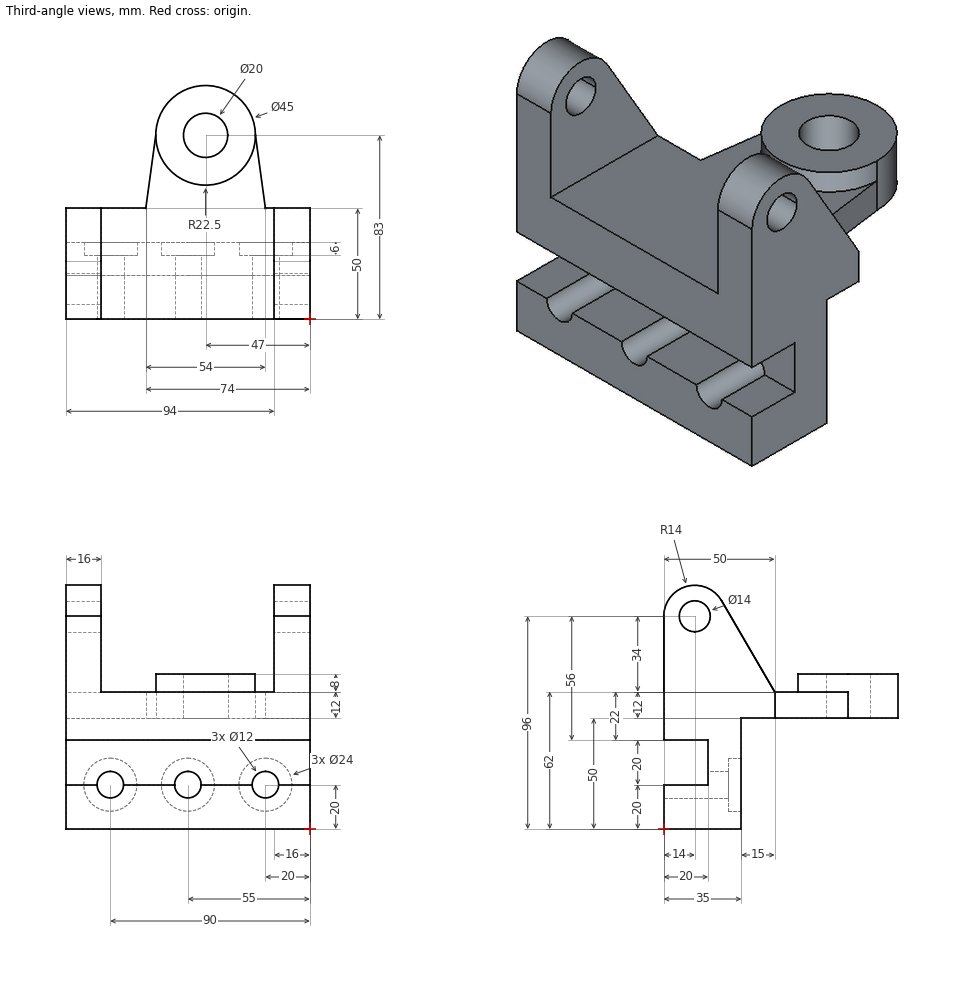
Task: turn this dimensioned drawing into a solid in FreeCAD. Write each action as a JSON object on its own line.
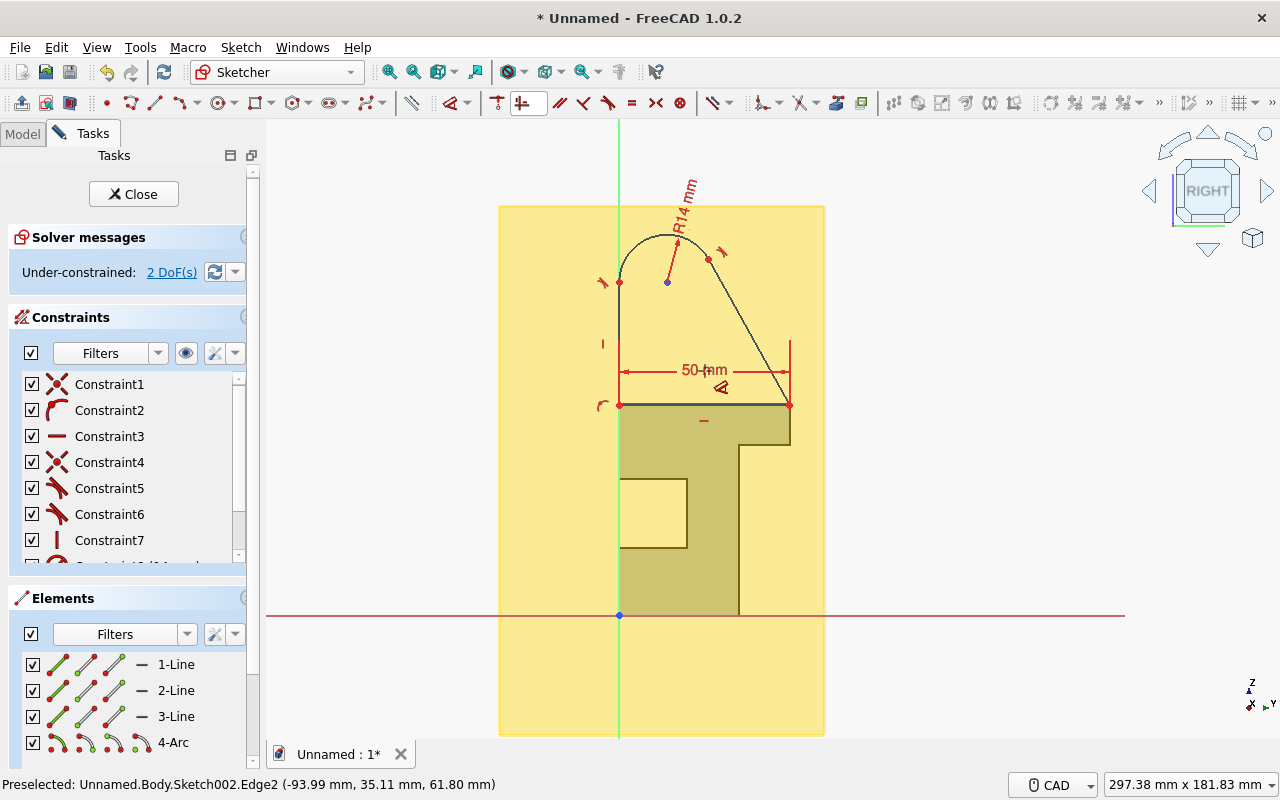
{"action": "left_click", "coordinate": [619, 368]}
{"action": "left_click", "coordinate": [585, 344]}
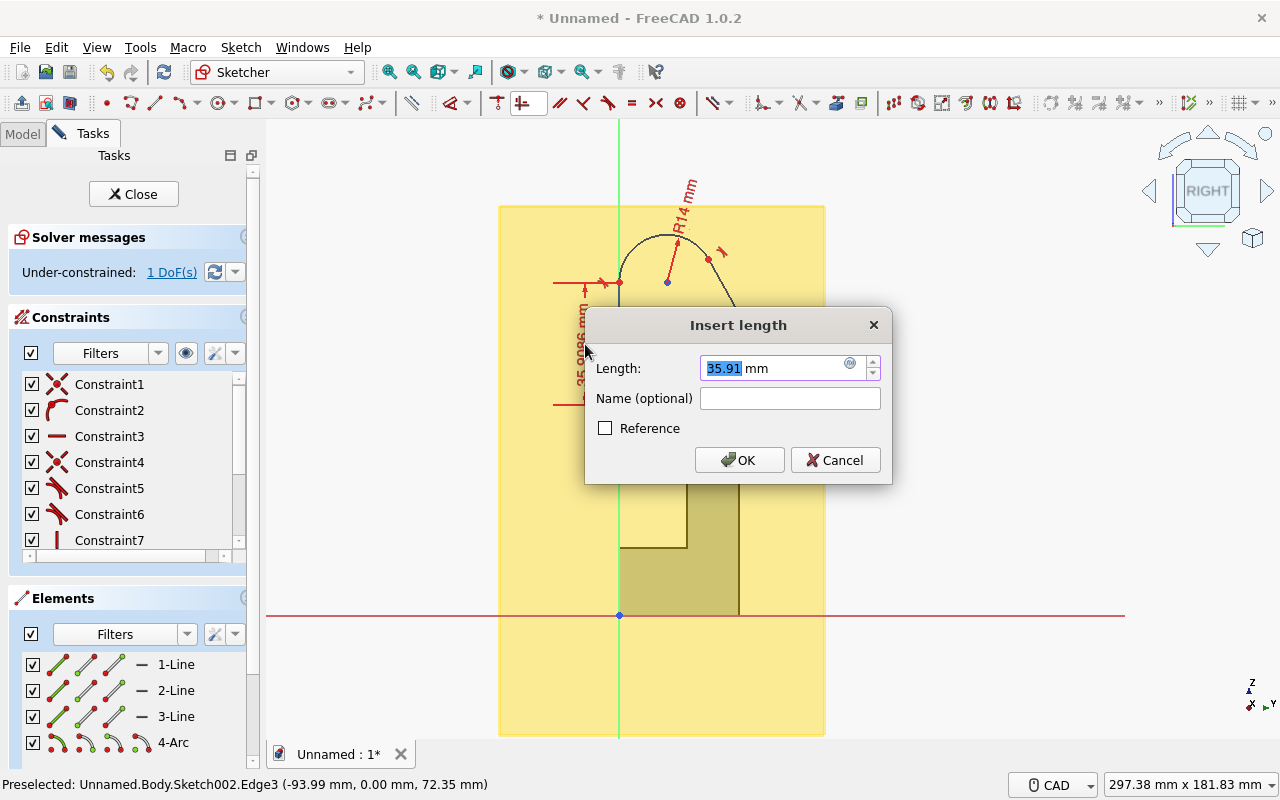
{"action": "type", "text": "34"}
{"action": "key", "text": "Return"}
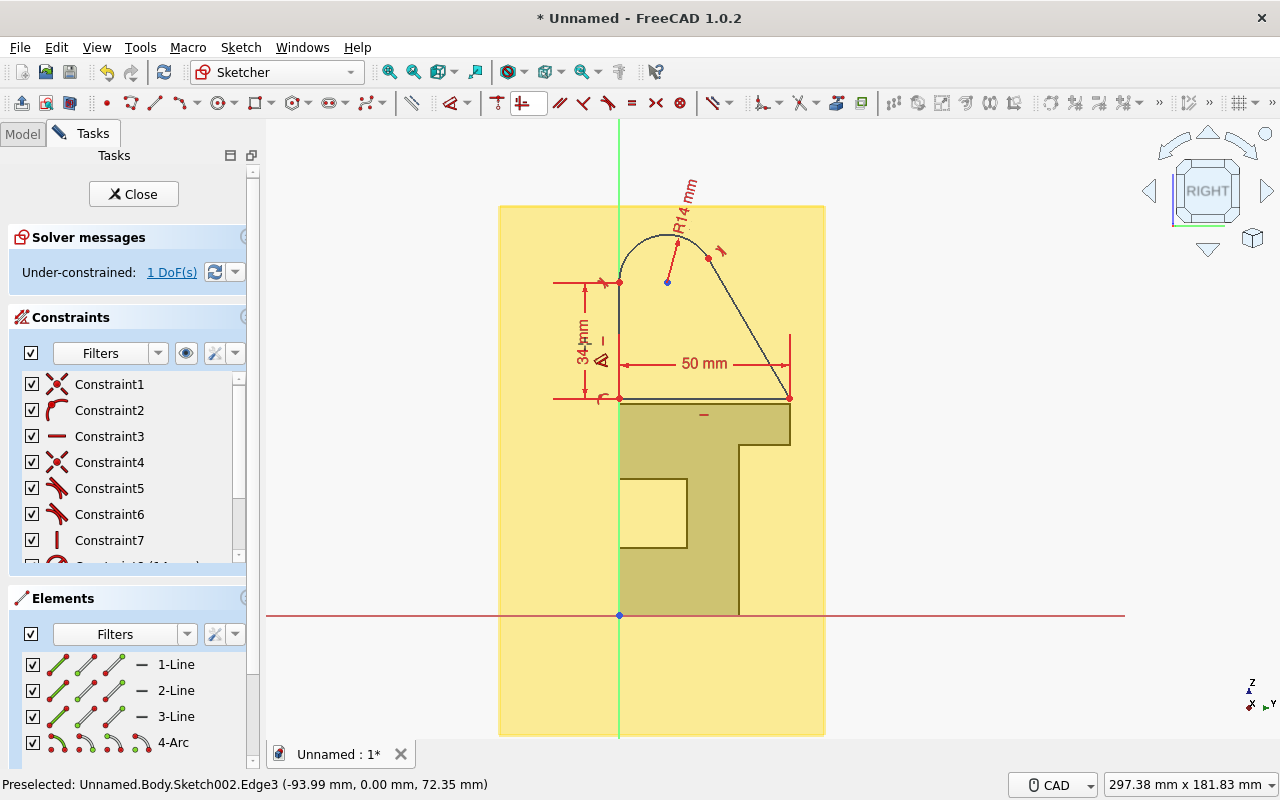
{"action": "left_click", "coordinate": [790, 399]}
{"action": "left_click", "coordinate": [824, 507]}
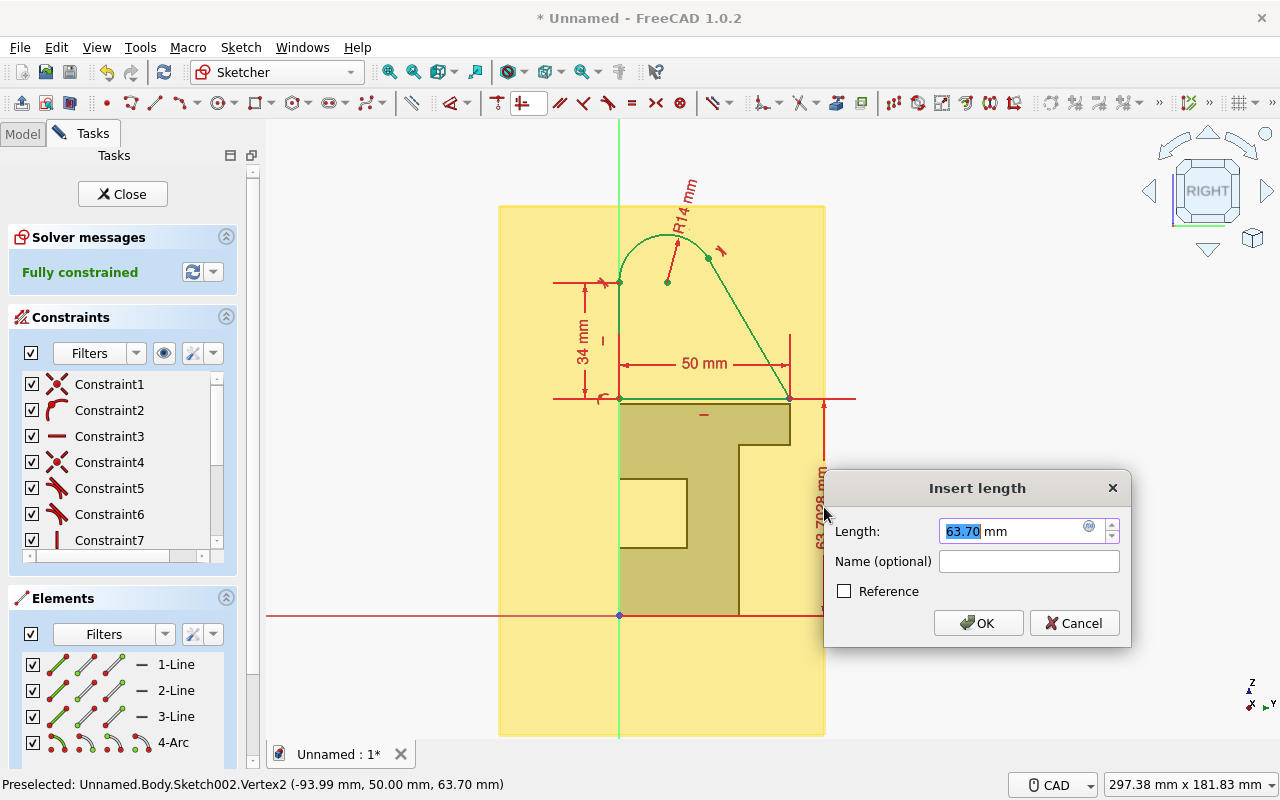
{"action": "type", "text": "62"}
{"action": "key", "text": "Return"}
{"action": "key", "text": "Escape"}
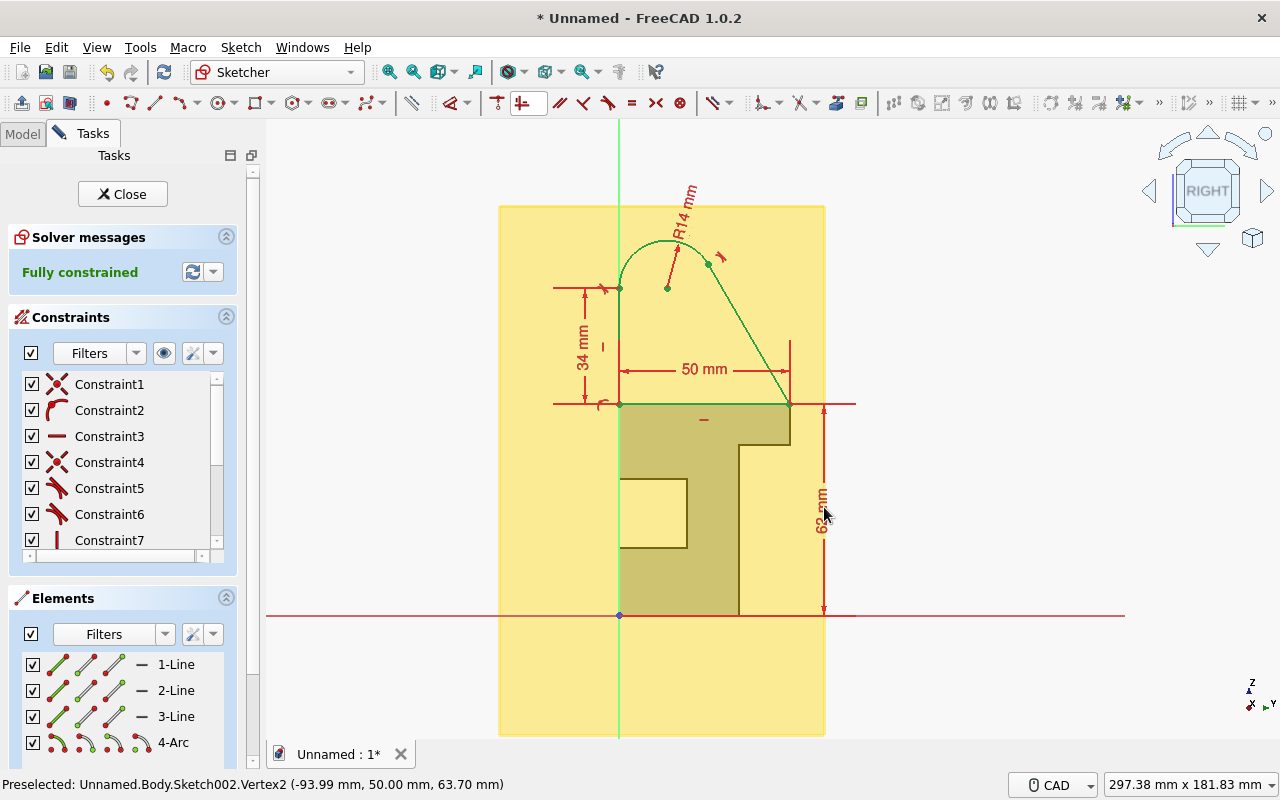
{"action": "left_click", "coordinate": [123, 194]}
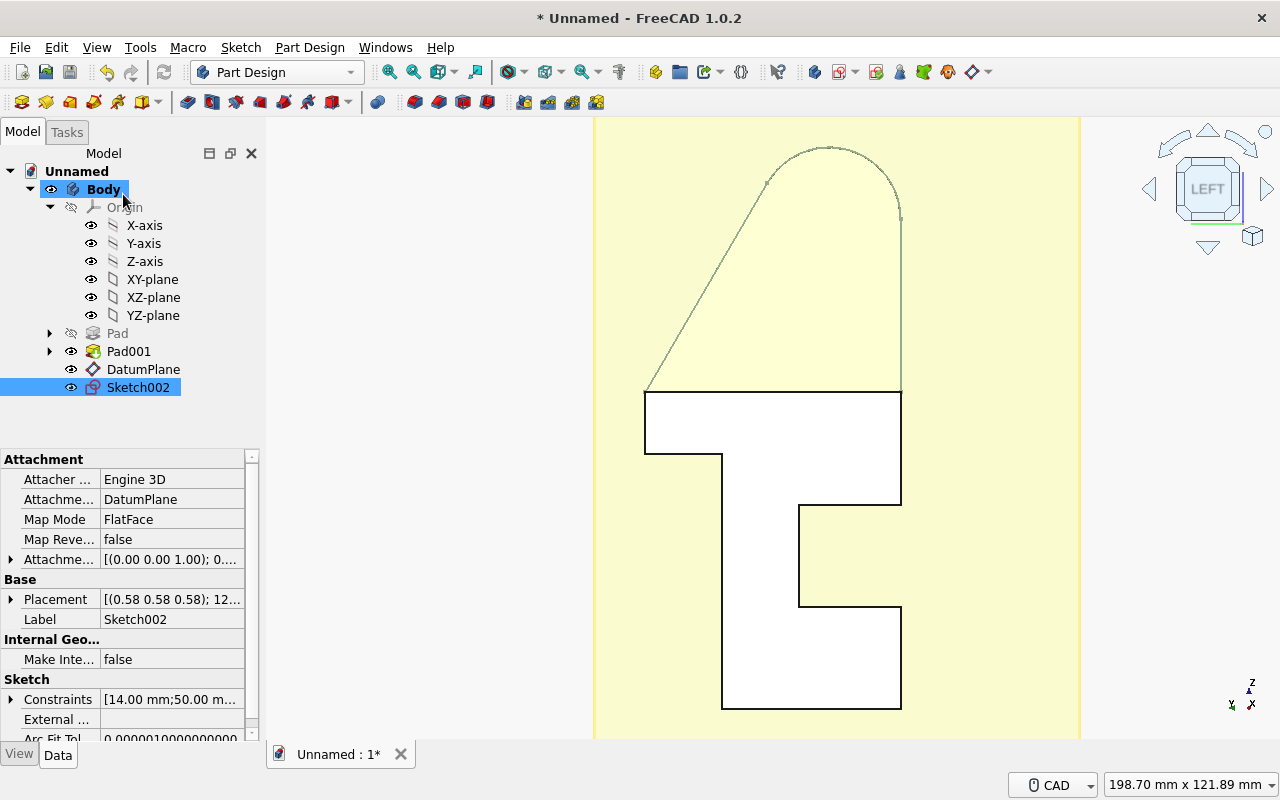
{"action": "left_click", "coordinate": [22, 102]}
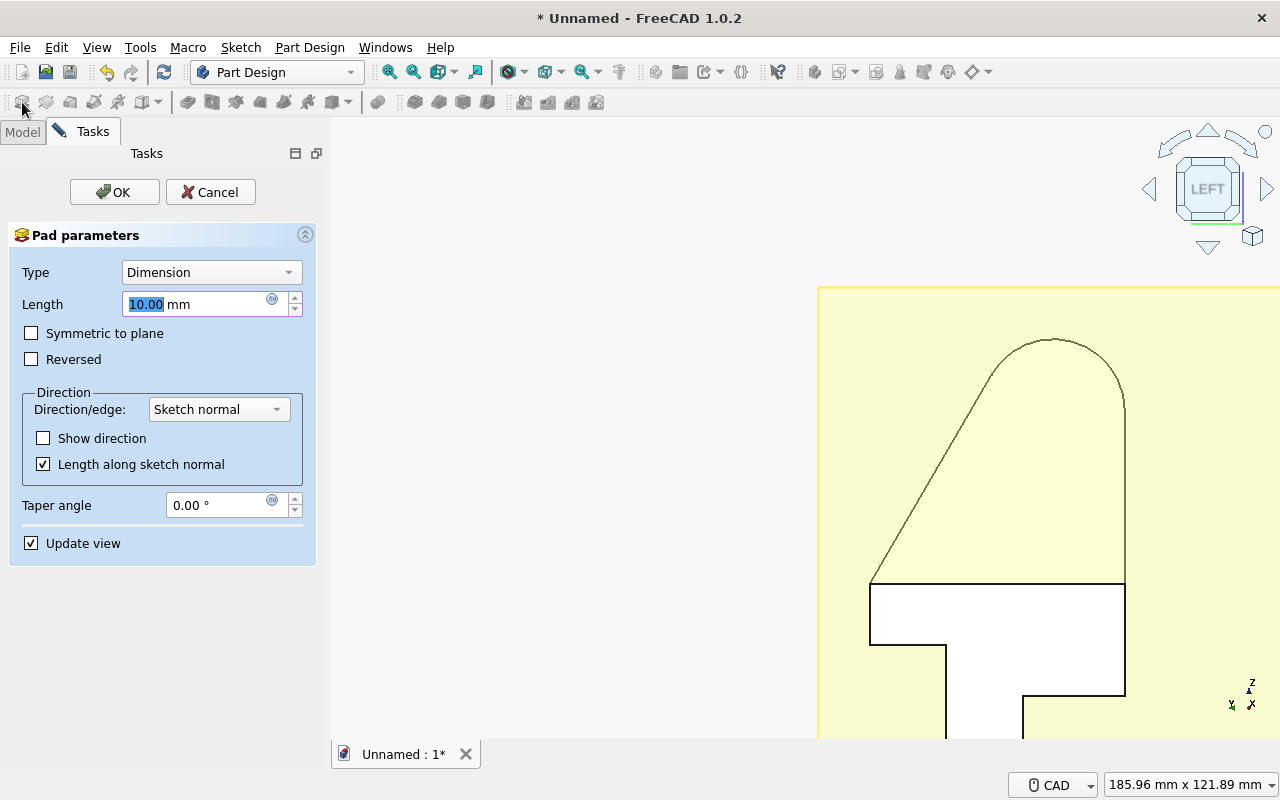
{"action": "type", "text": "16"}
{"action": "key", "text": "Tab"}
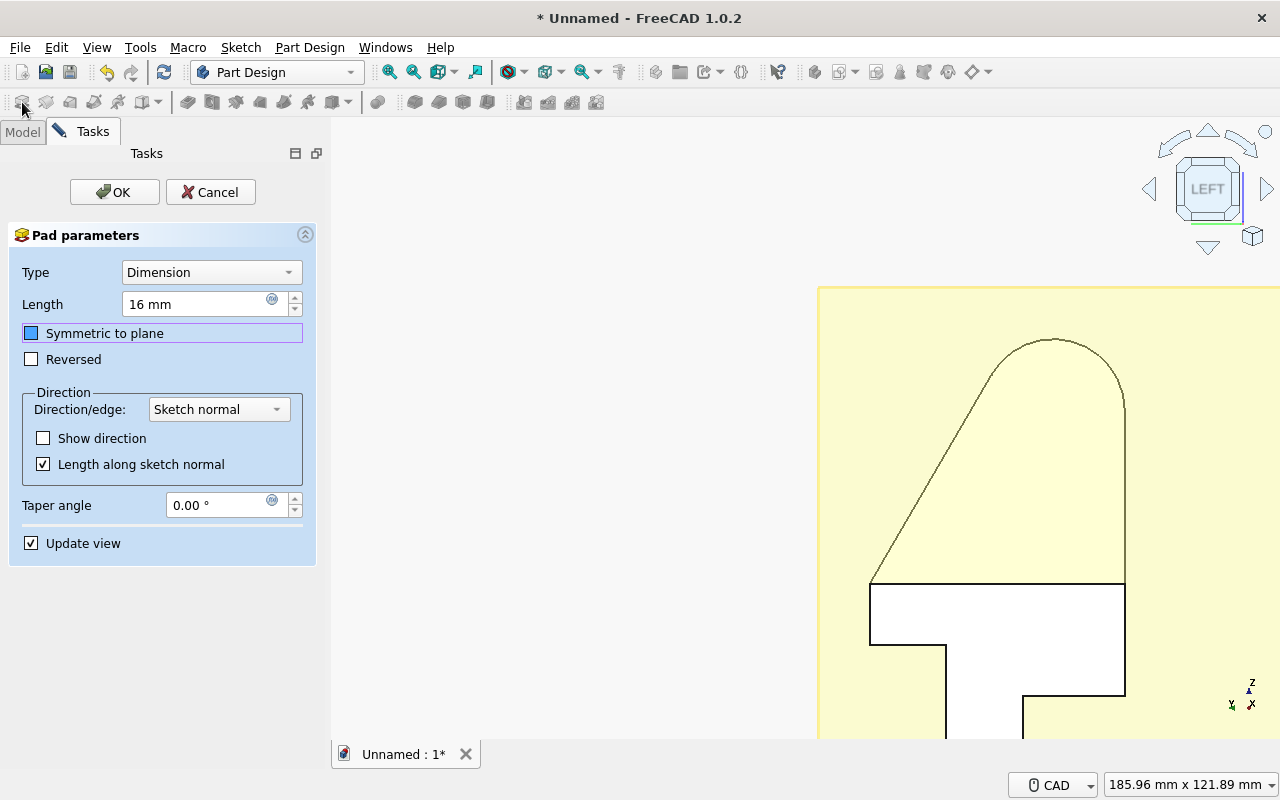
{"action": "left_click", "coordinate": [30, 359]}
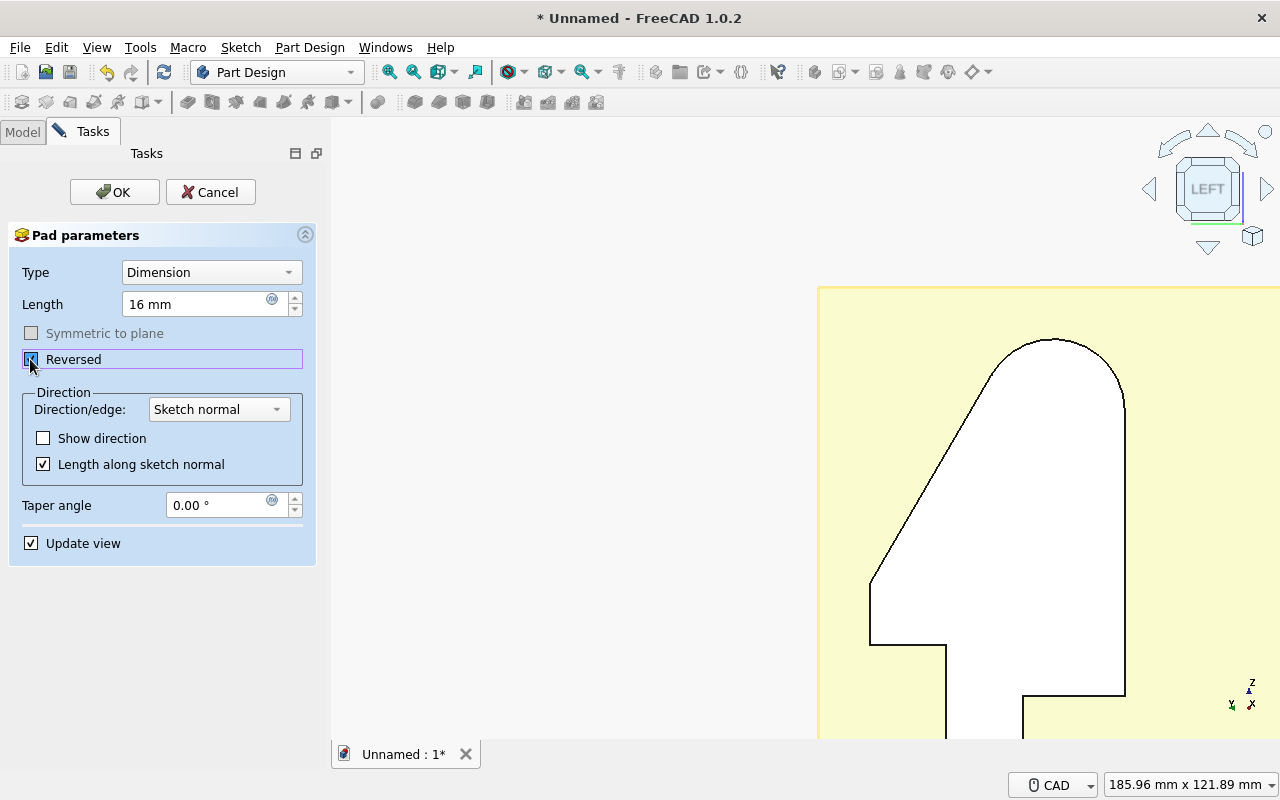
{"action": "left_click", "coordinate": [115, 192]}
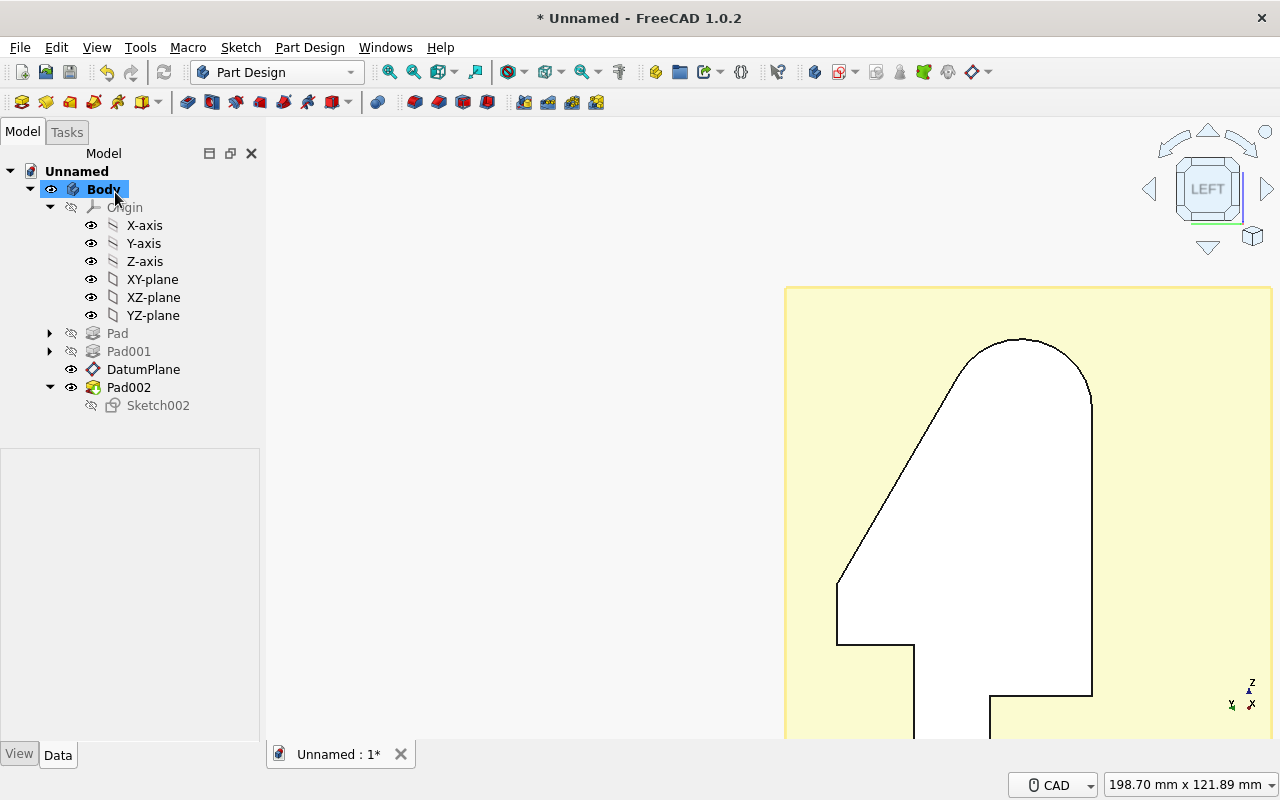
{"action": "left_click", "coordinate": [116, 369]}
{"action": "key", "text": "space"}